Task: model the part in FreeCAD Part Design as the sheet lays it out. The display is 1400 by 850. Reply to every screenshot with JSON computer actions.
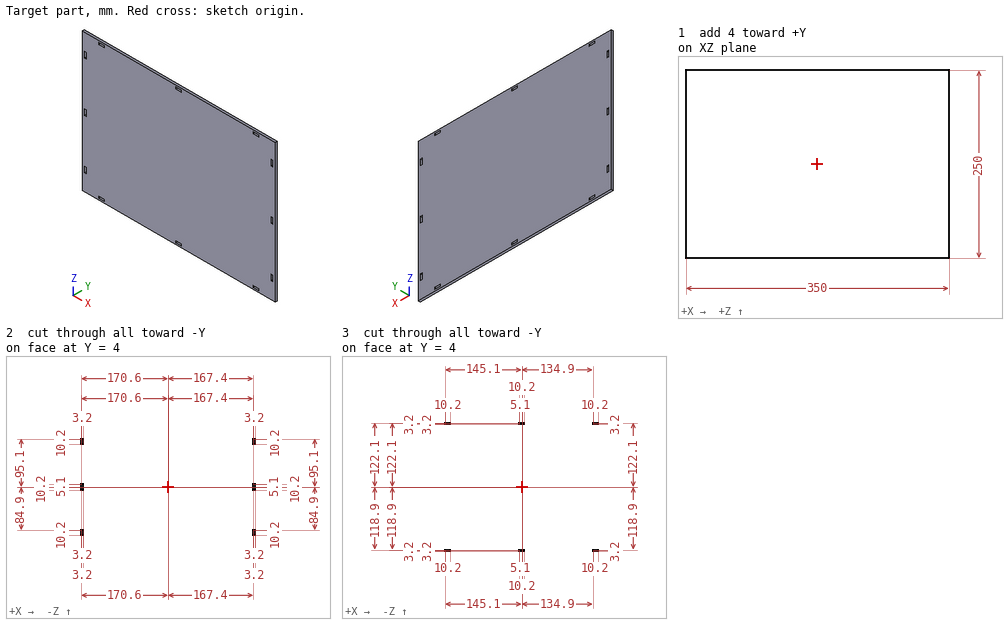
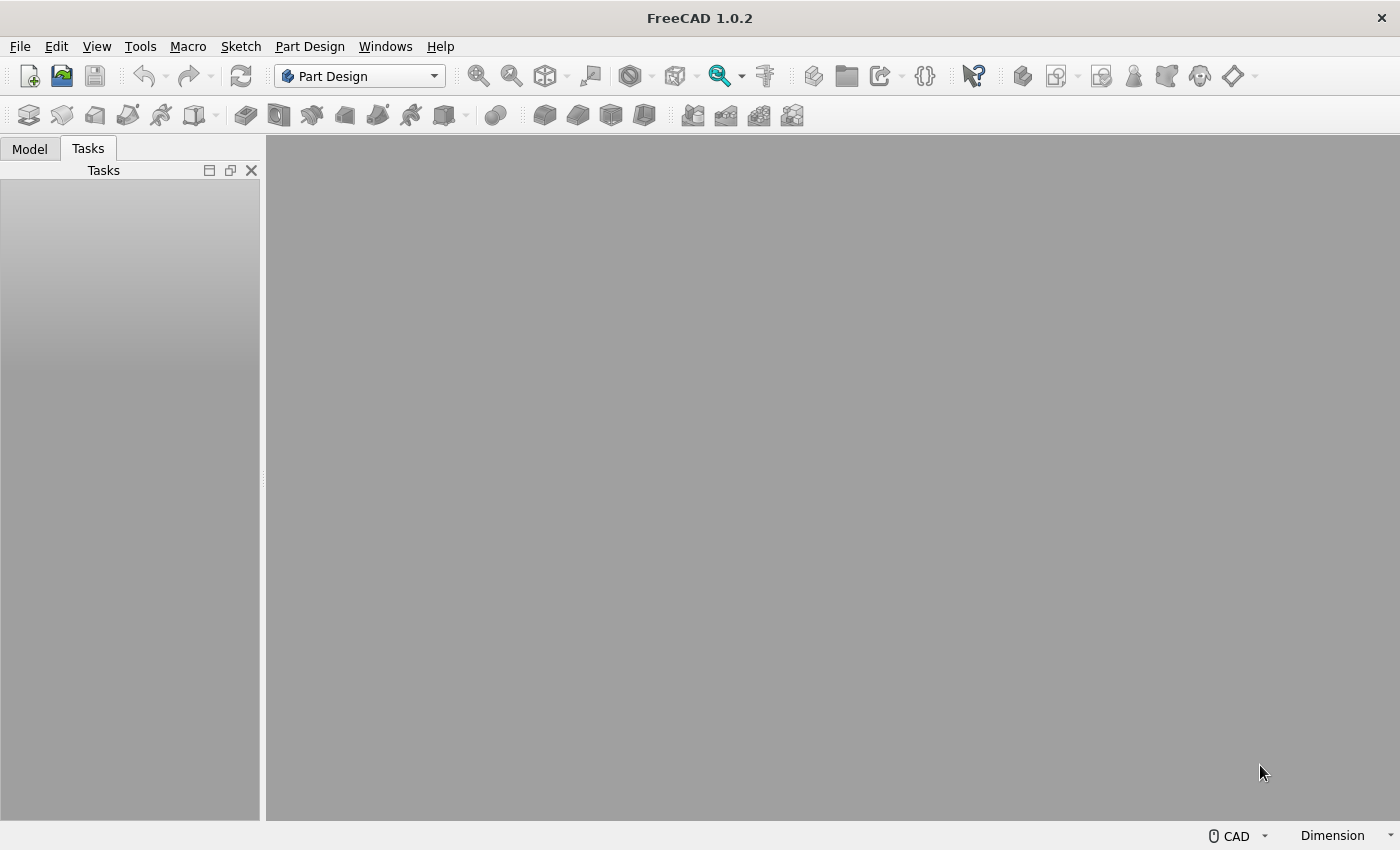
{"action": "left_click", "coordinate": [29, 76]}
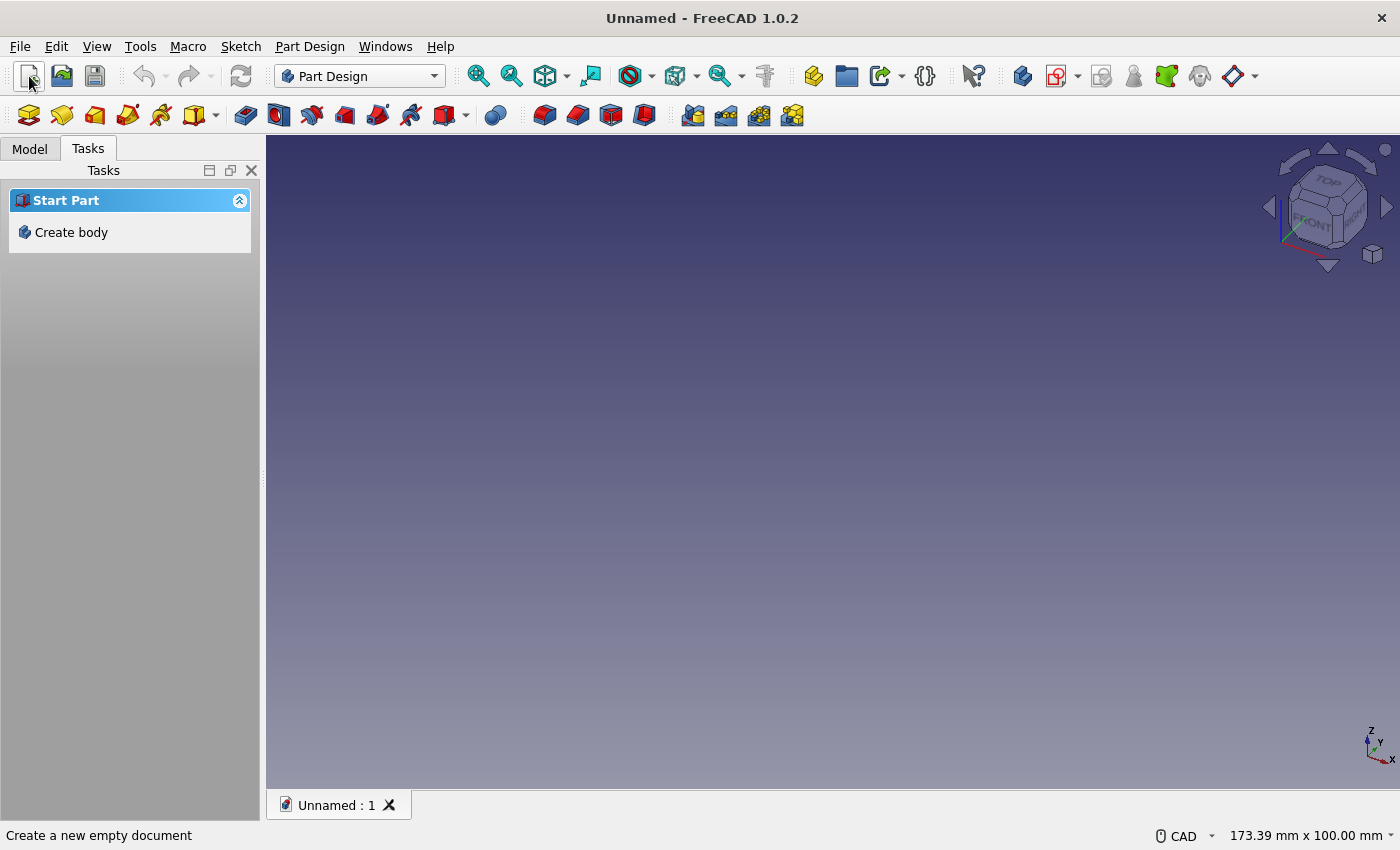
{"action": "left_click", "coordinate": [1056, 76]}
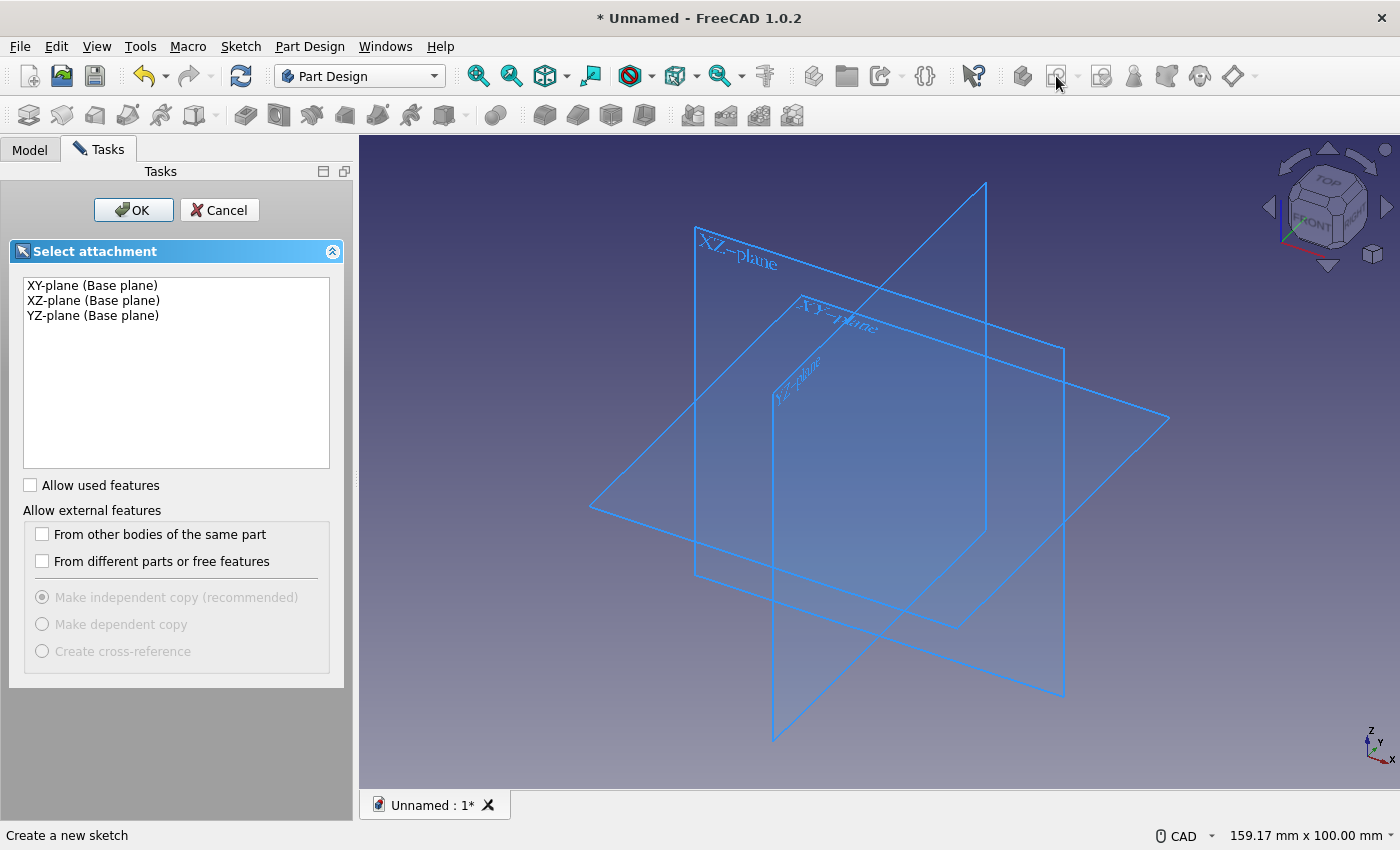
{"action": "left_click", "coordinate": [84, 300]}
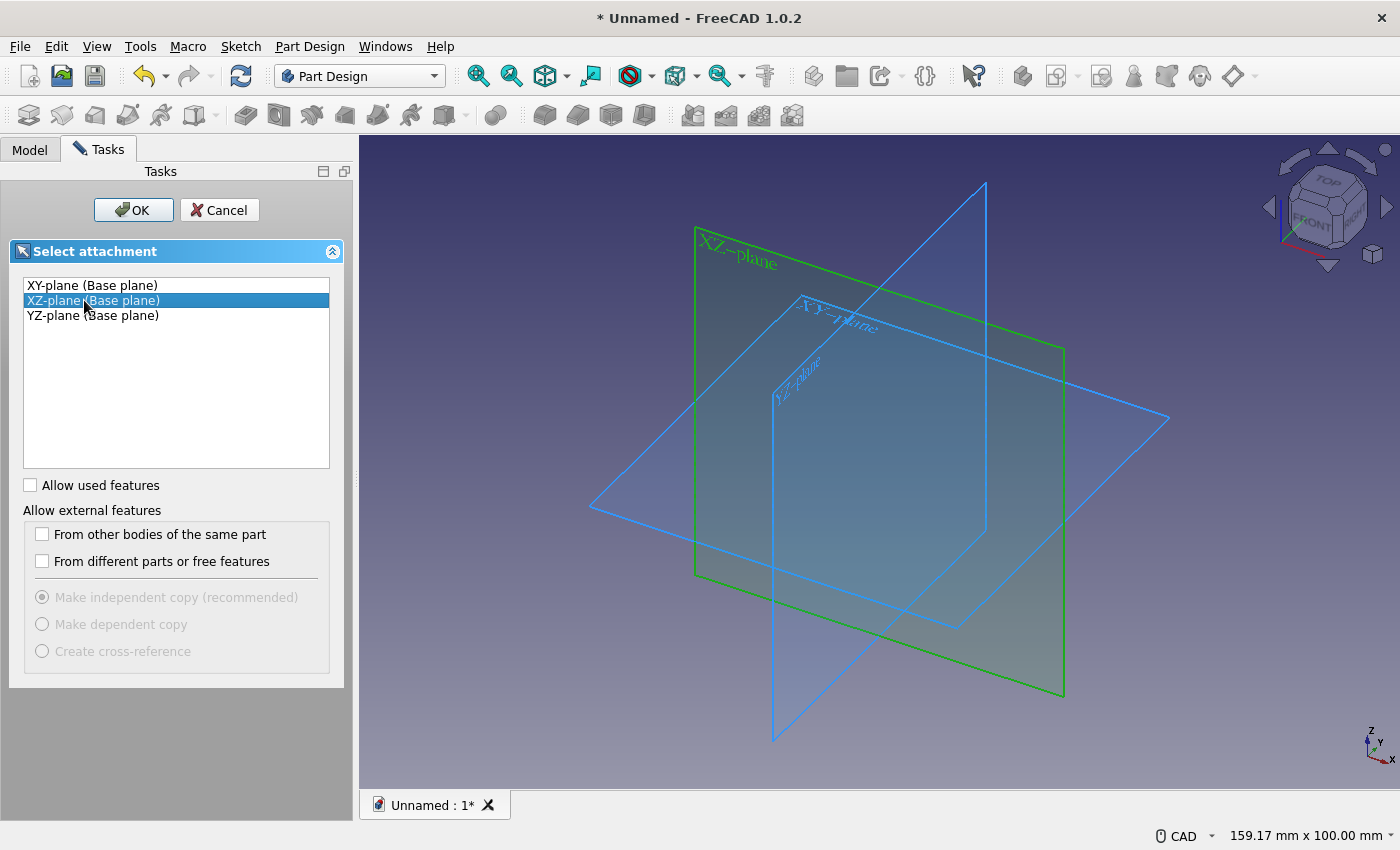
{"action": "left_click", "coordinate": [134, 210]}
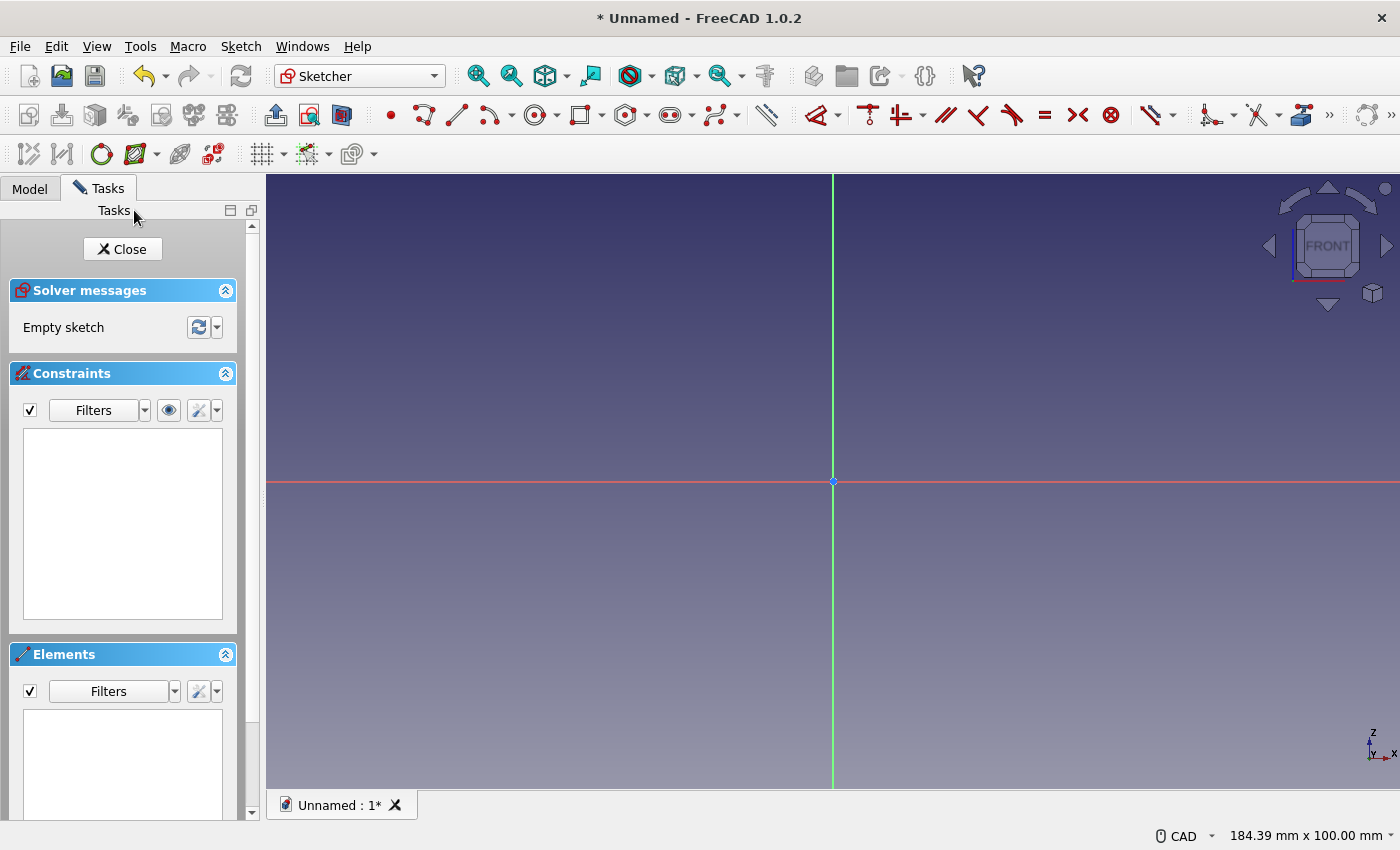
{"action": "scroll", "coordinate": [742, 482], "scroll_direction": "down", "scroll_amount": 7}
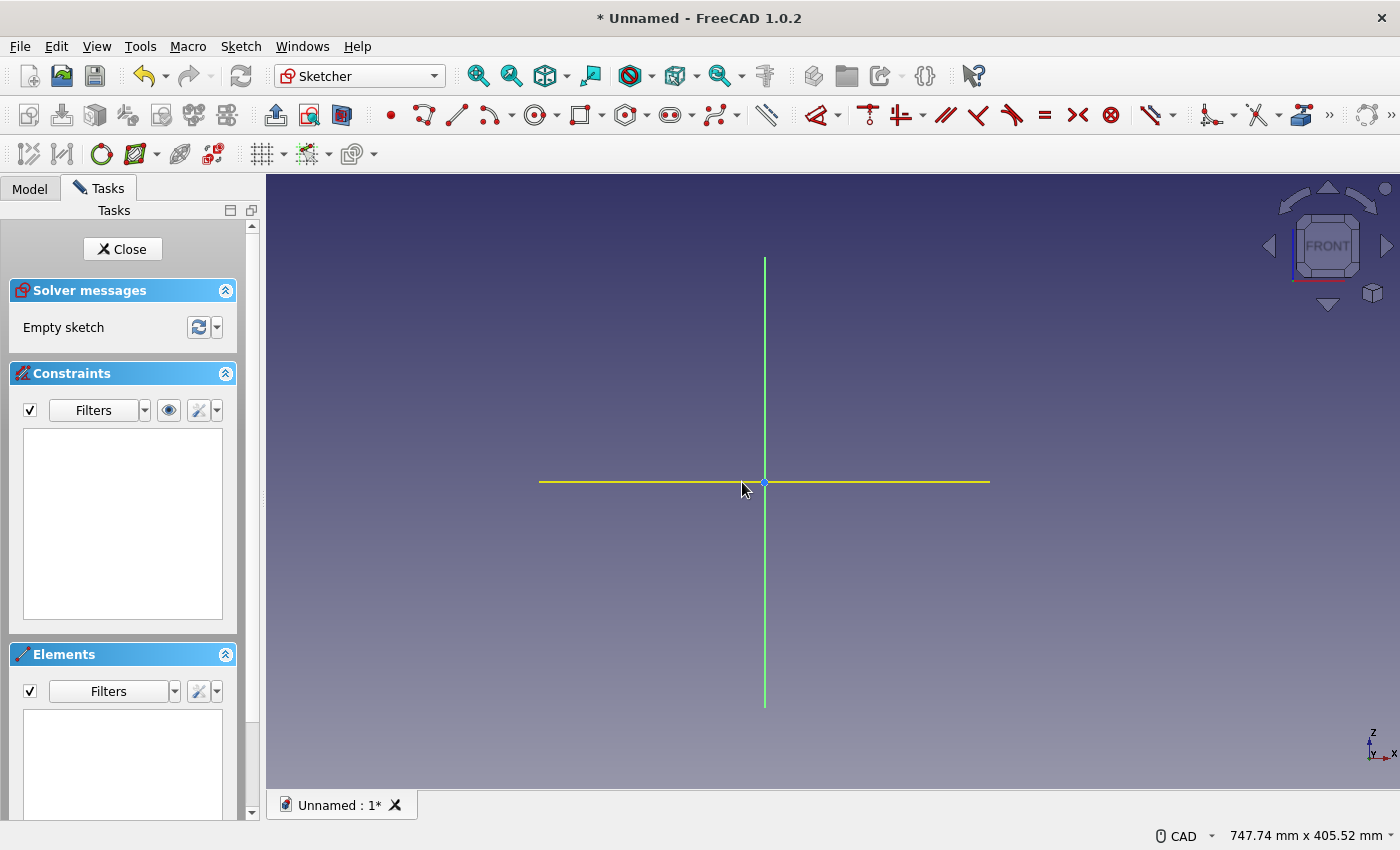
{"action": "key", "text": "g v"}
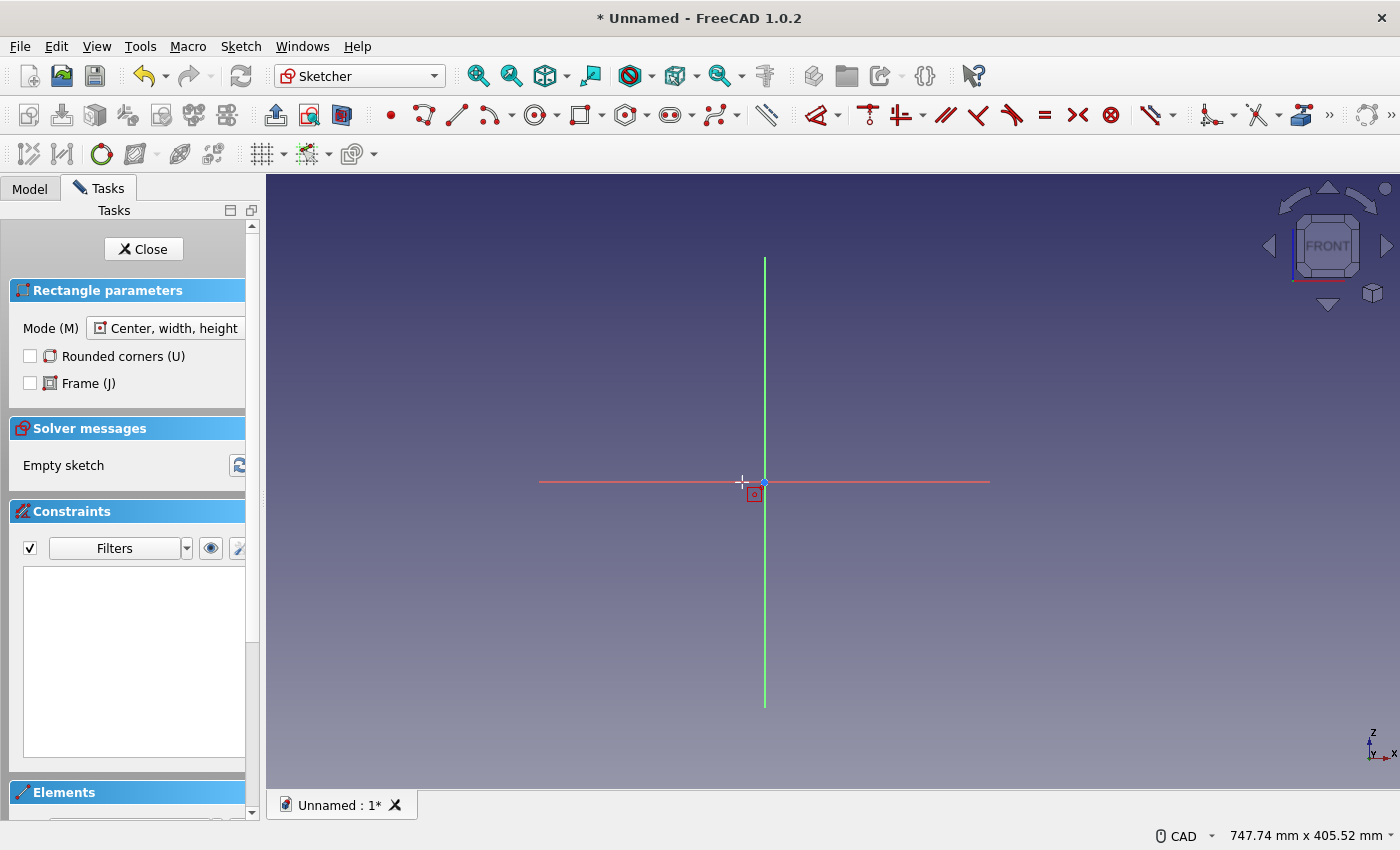
{"action": "left_click", "coordinate": [765, 482]}
{"action": "left_click", "coordinate": [1030, 293]}
{"action": "key", "text": "Escape"}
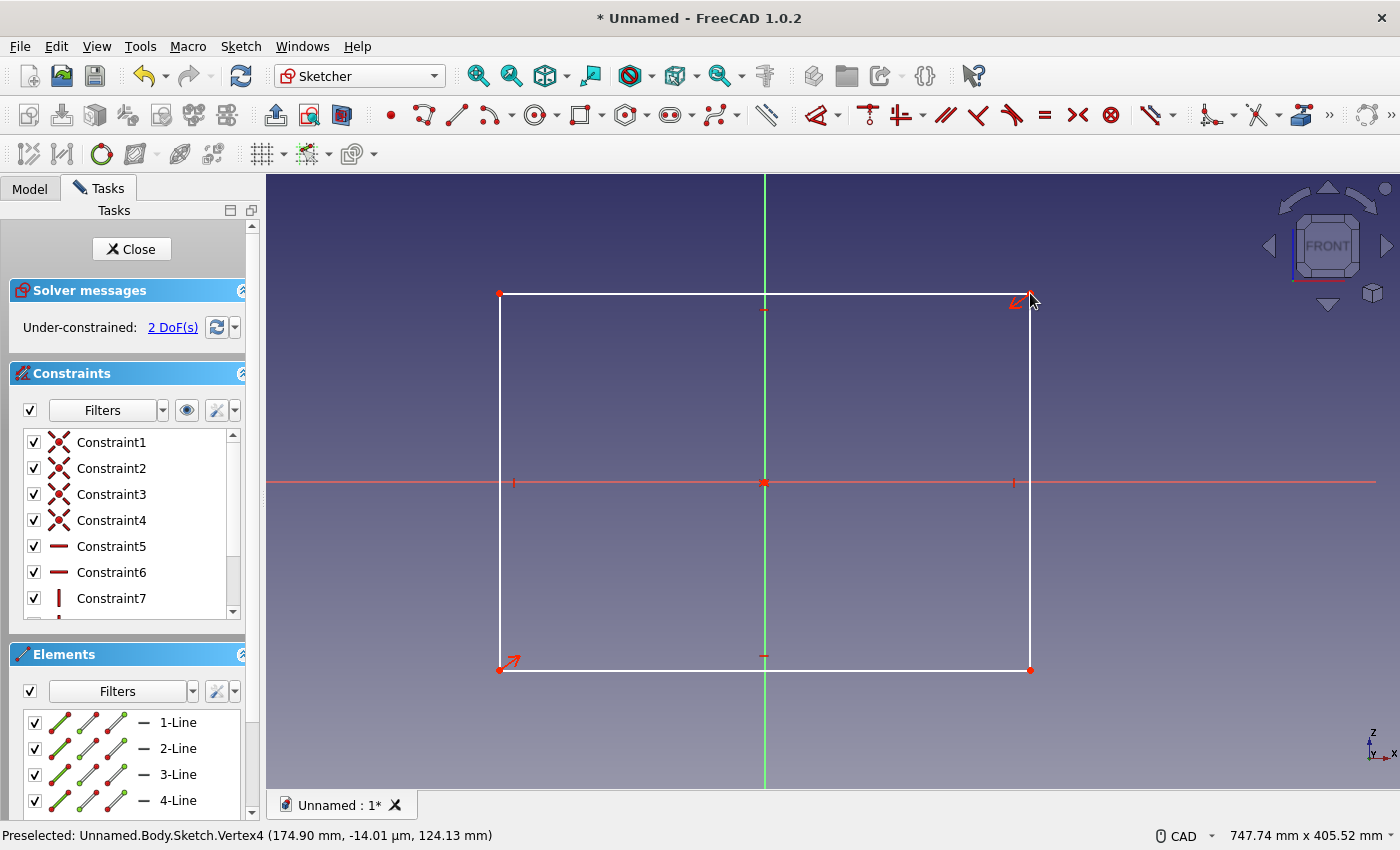
{"action": "left_click", "coordinate": [816, 116]}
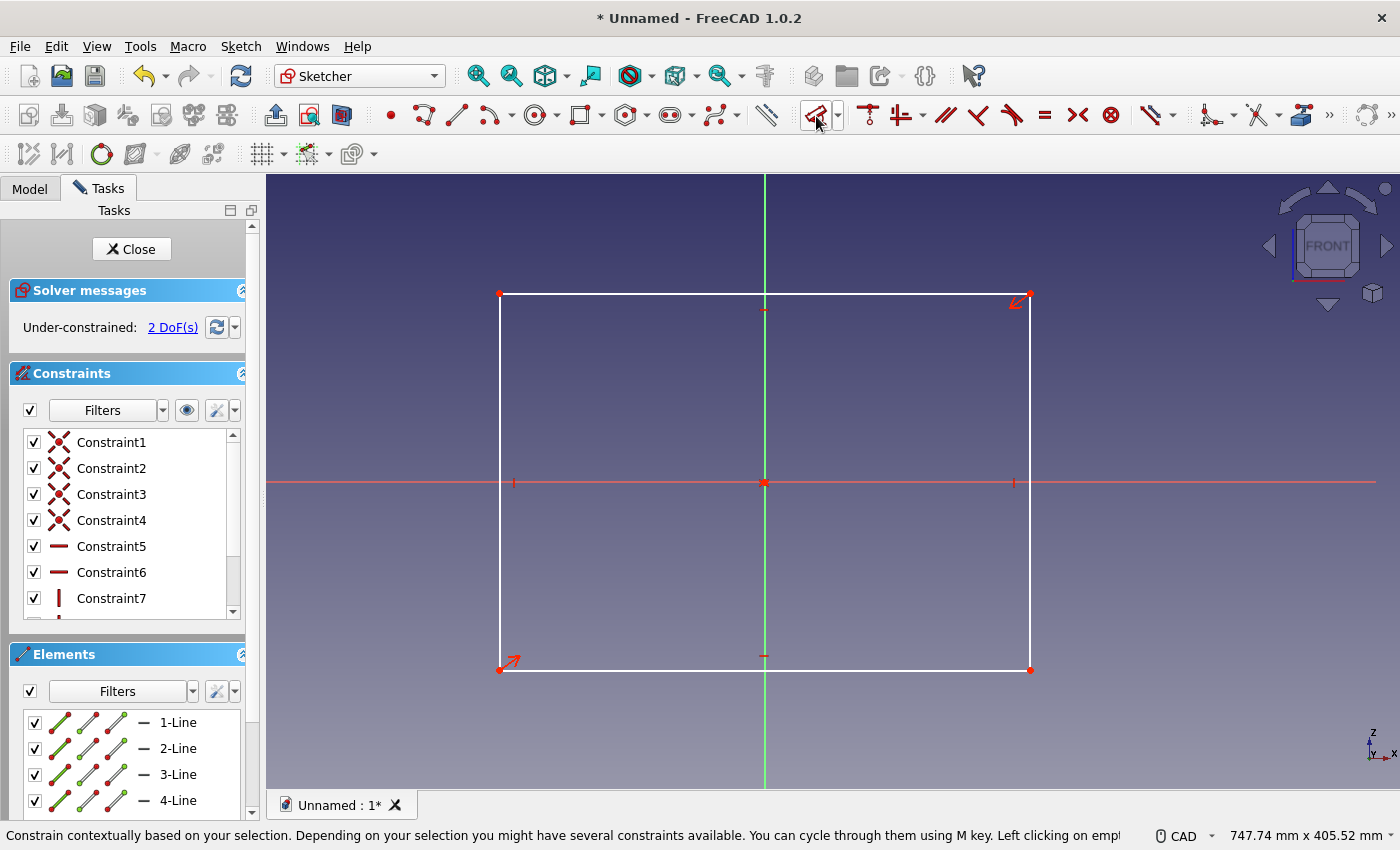
{"action": "left_click", "coordinate": [659, 671]}
{"action": "left_click", "coordinate": [643, 705]}